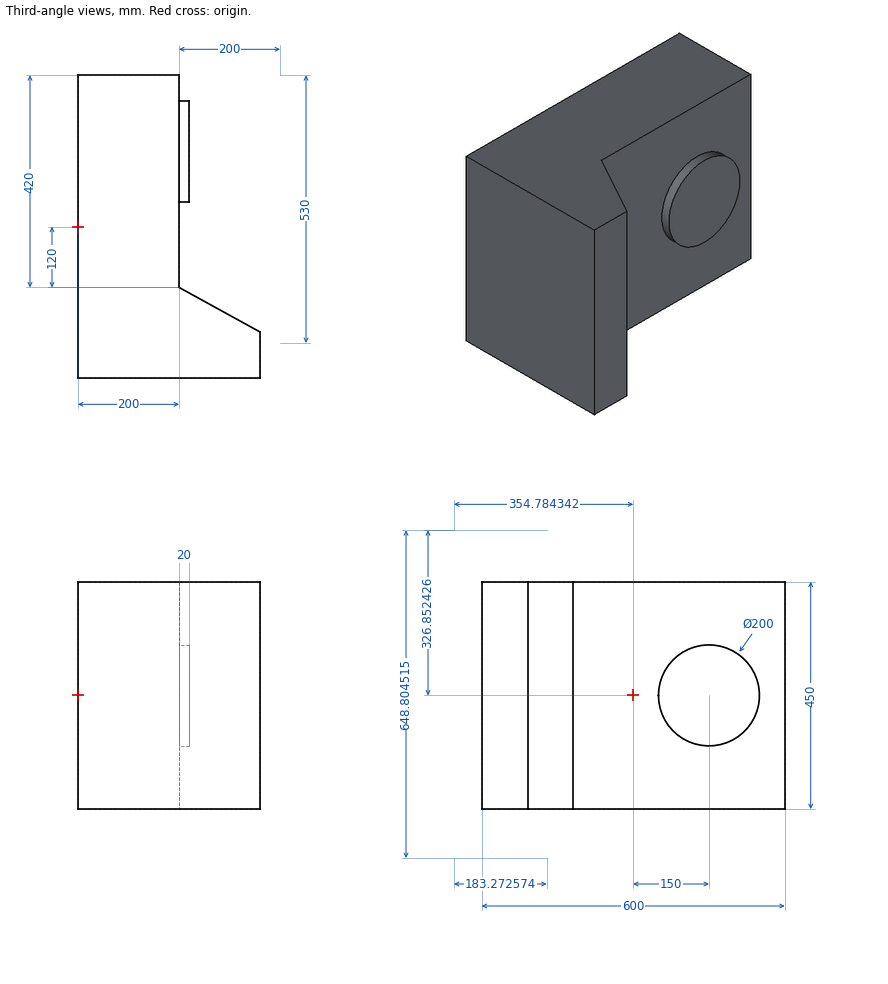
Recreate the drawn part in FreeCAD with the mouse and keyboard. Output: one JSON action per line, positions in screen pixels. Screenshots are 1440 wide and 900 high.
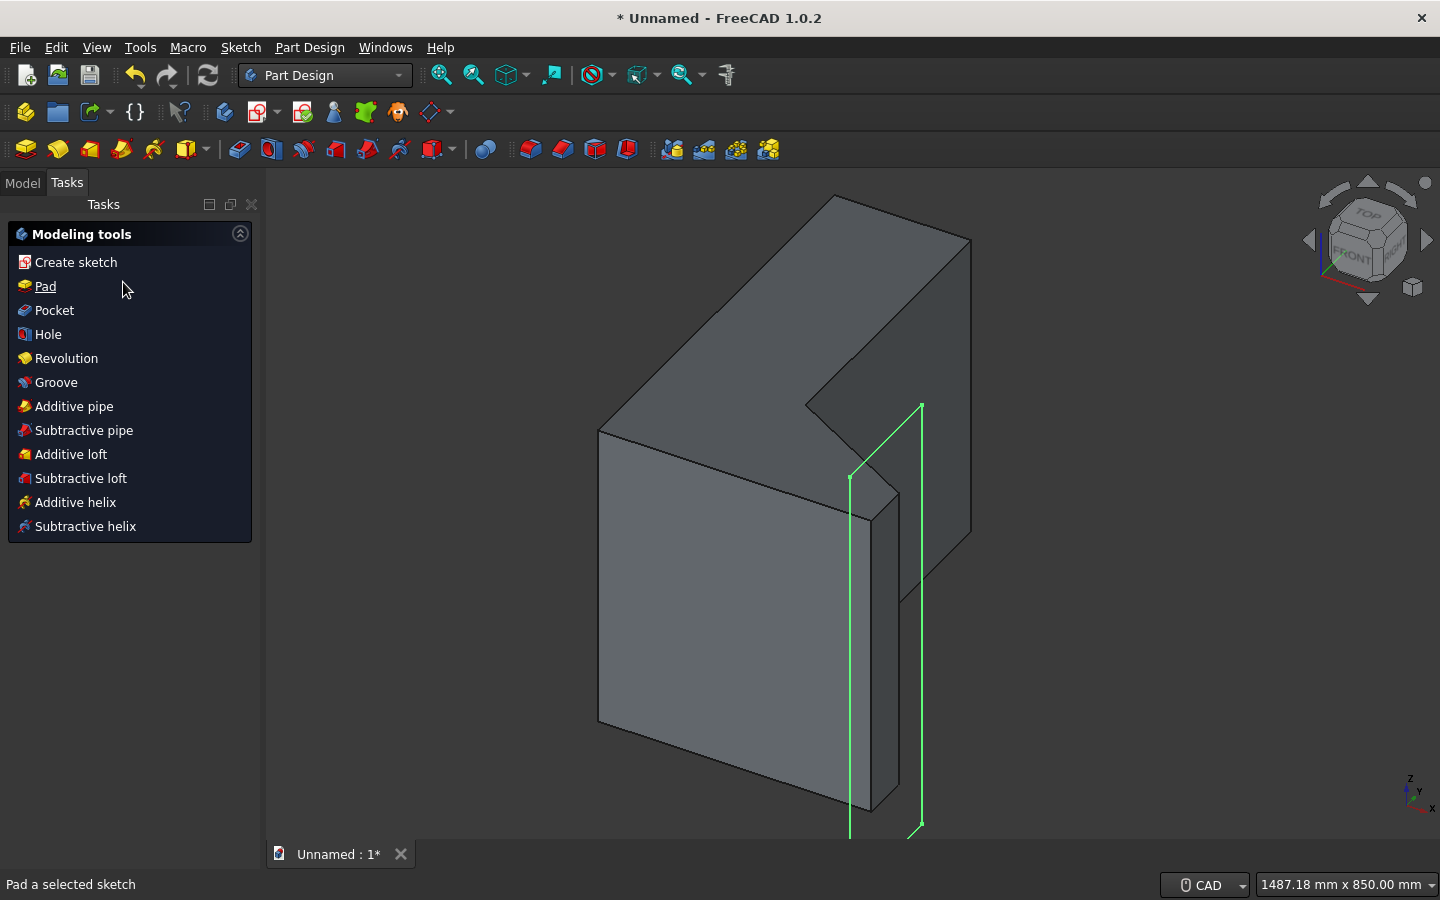
{"action": "left_click", "coordinate": [240, 150]}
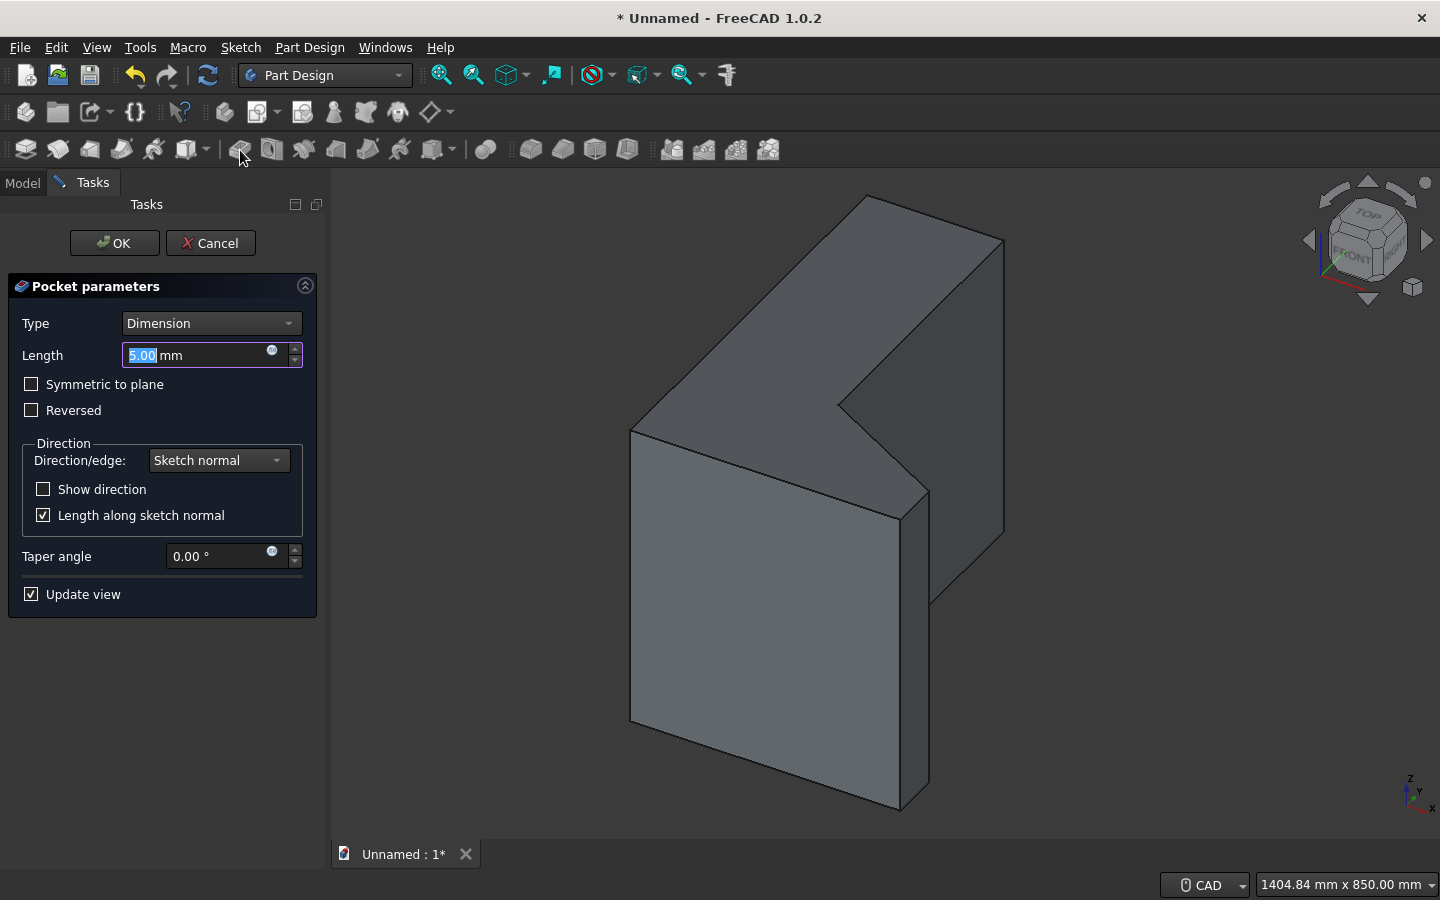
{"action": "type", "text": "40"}
{"action": "key", "text": "Tab"}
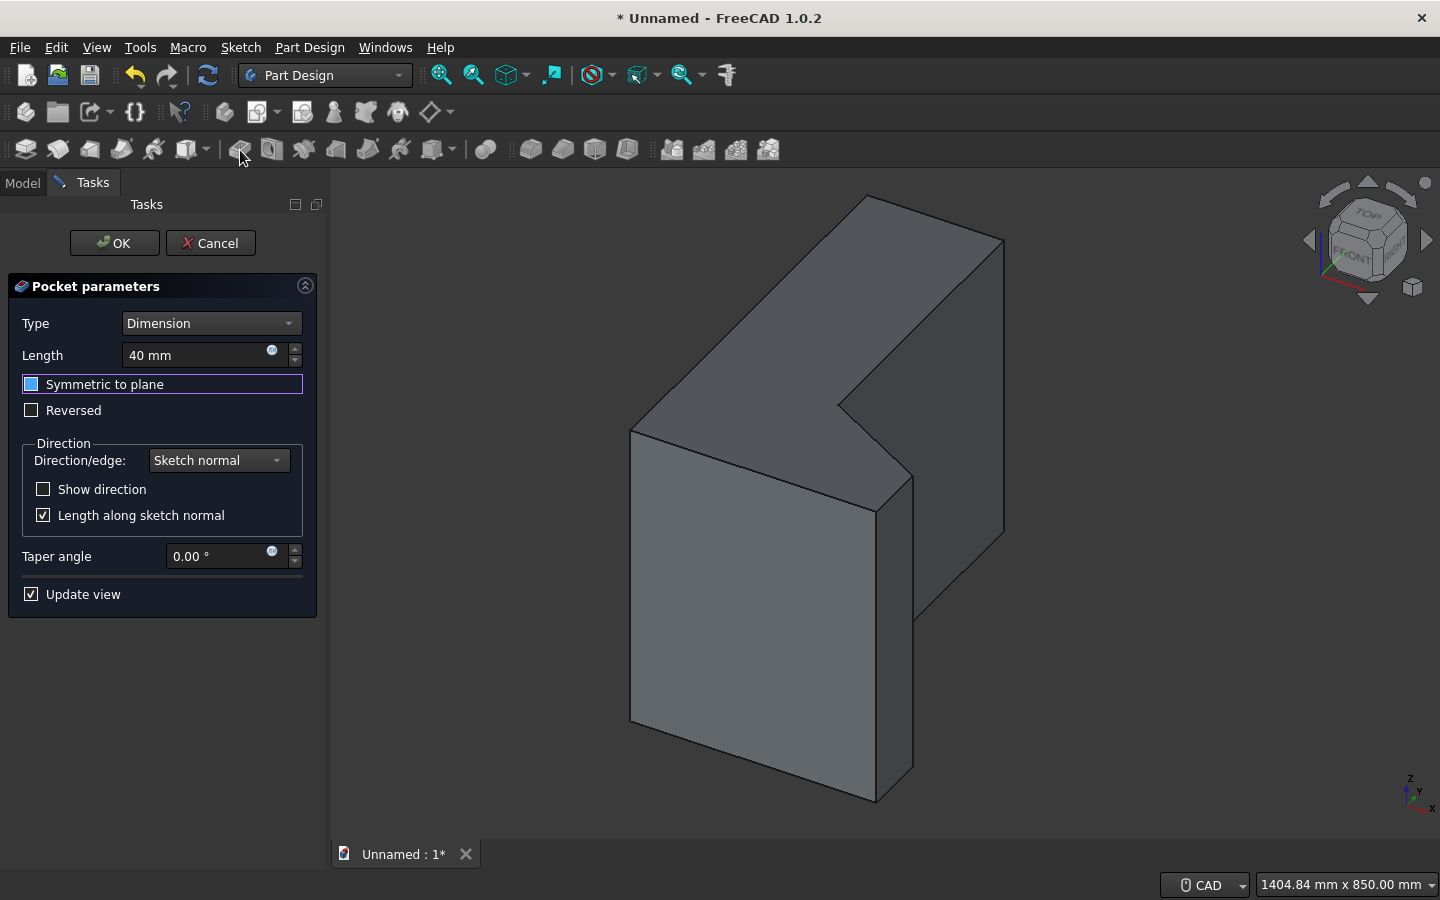
{"action": "left_click", "coordinate": [115, 243]}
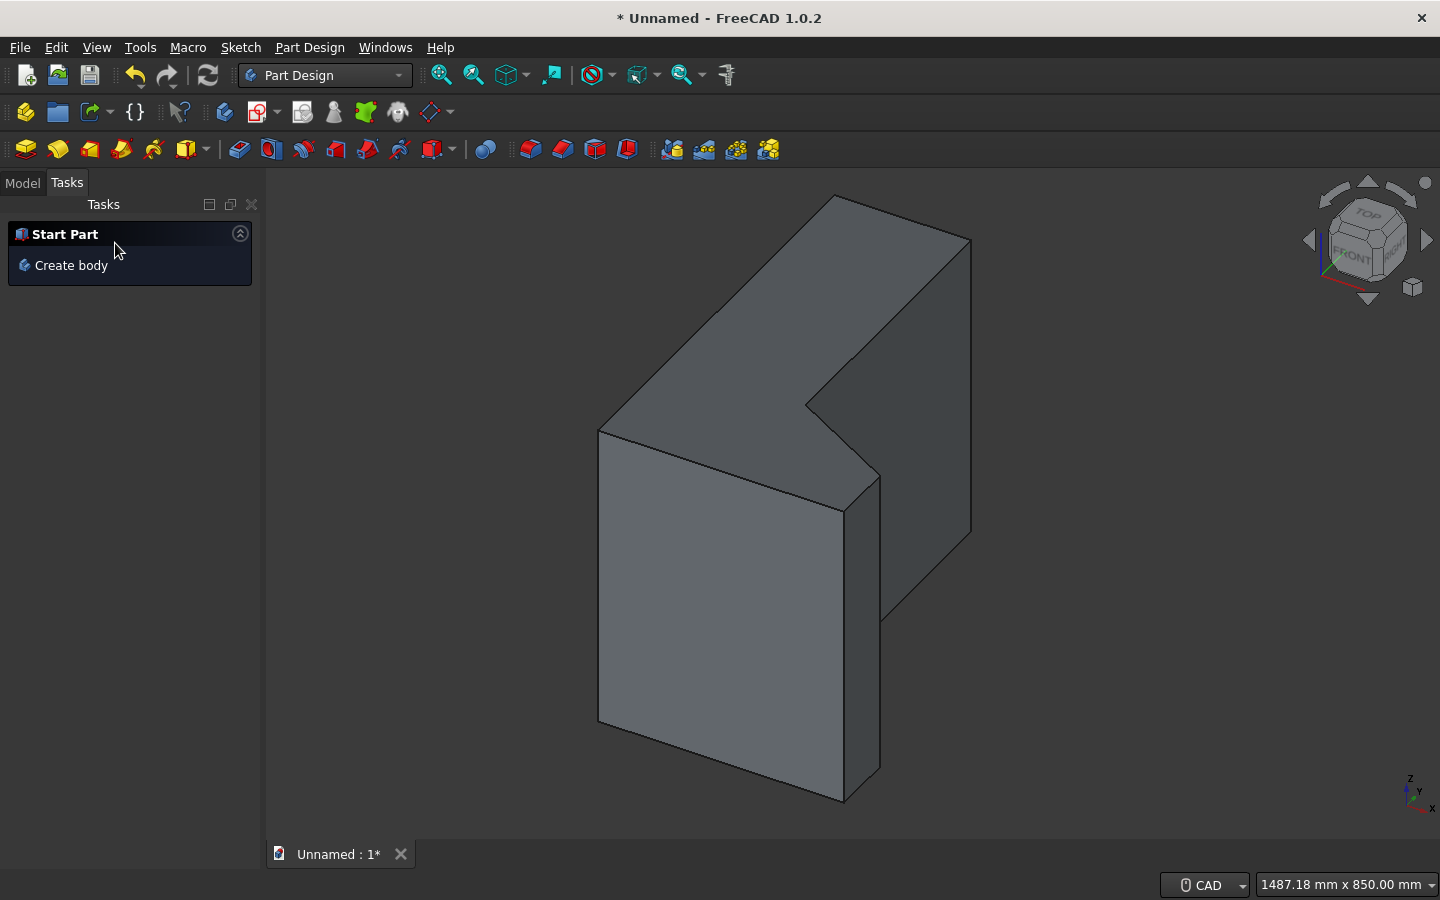
{"action": "left_click", "coordinate": [889, 467]}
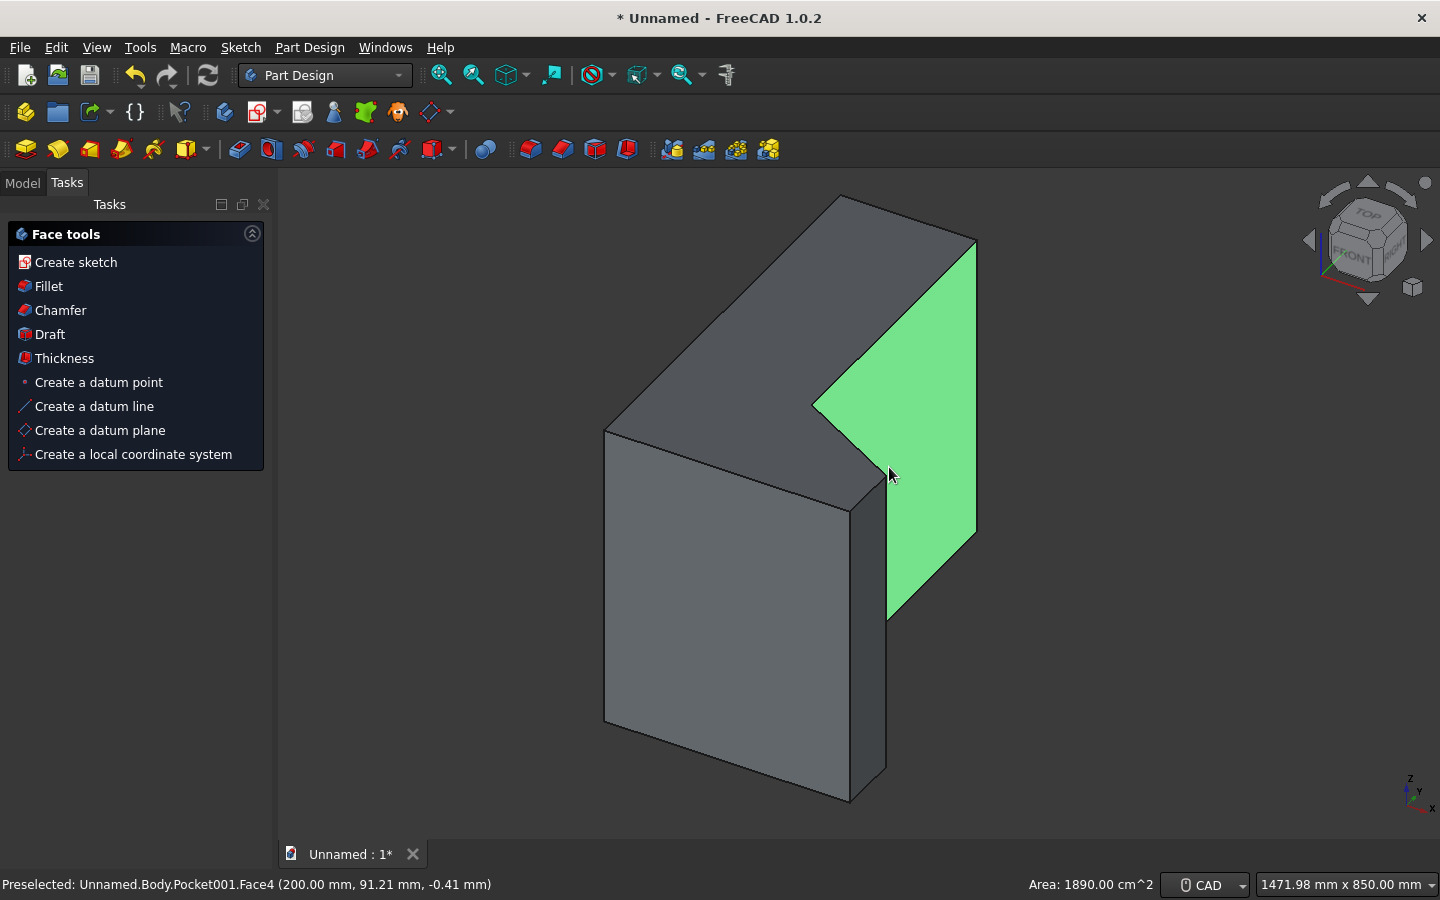
{"action": "left_click", "coordinate": [258, 112]}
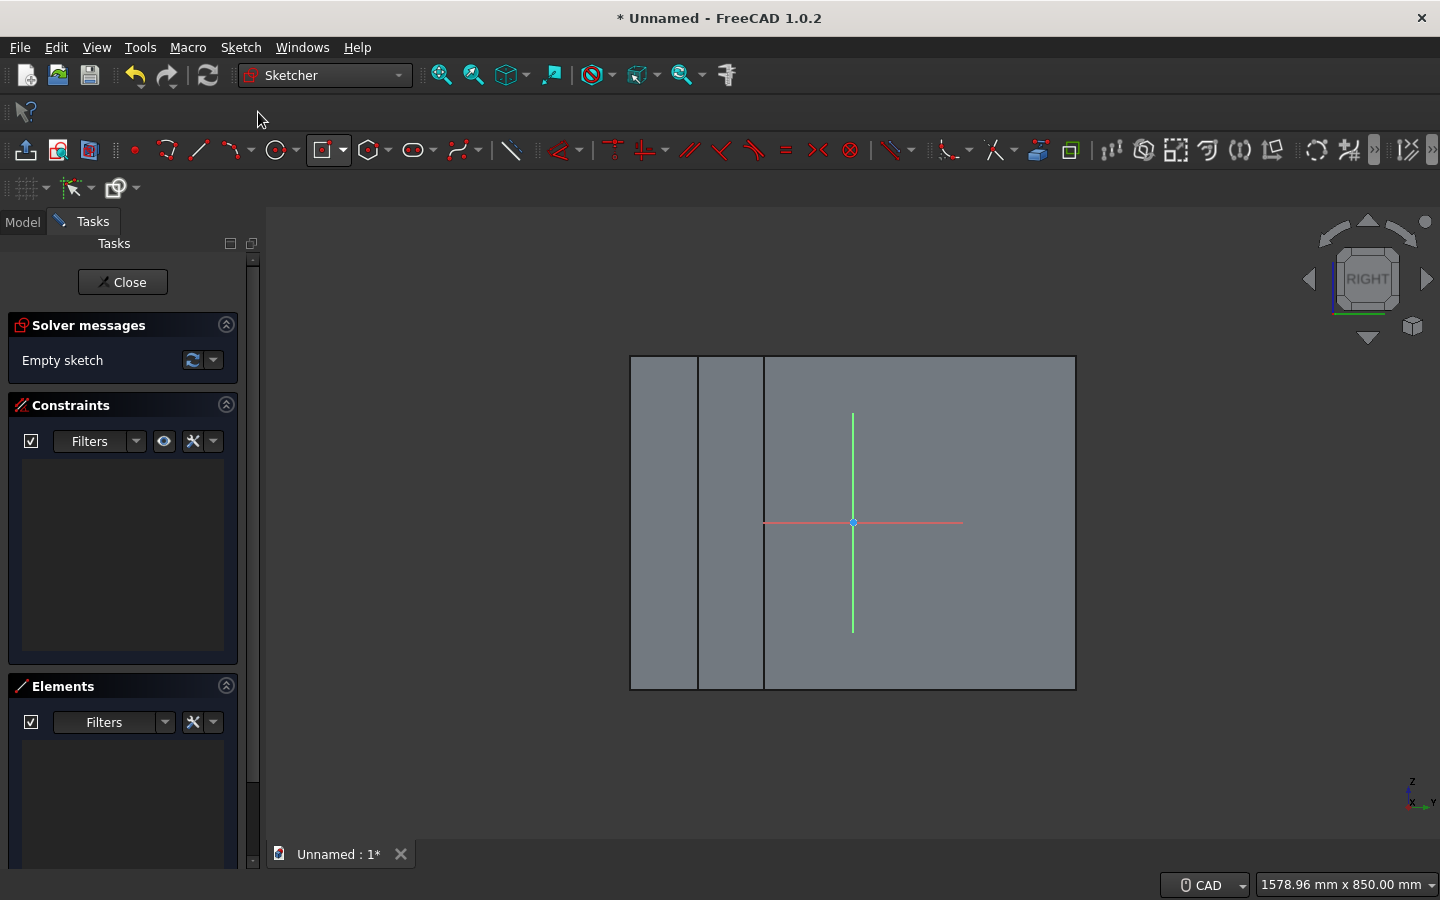
{"action": "scroll", "coordinate": [1040, 523], "scroll_direction": "up", "scroll_amount": 5}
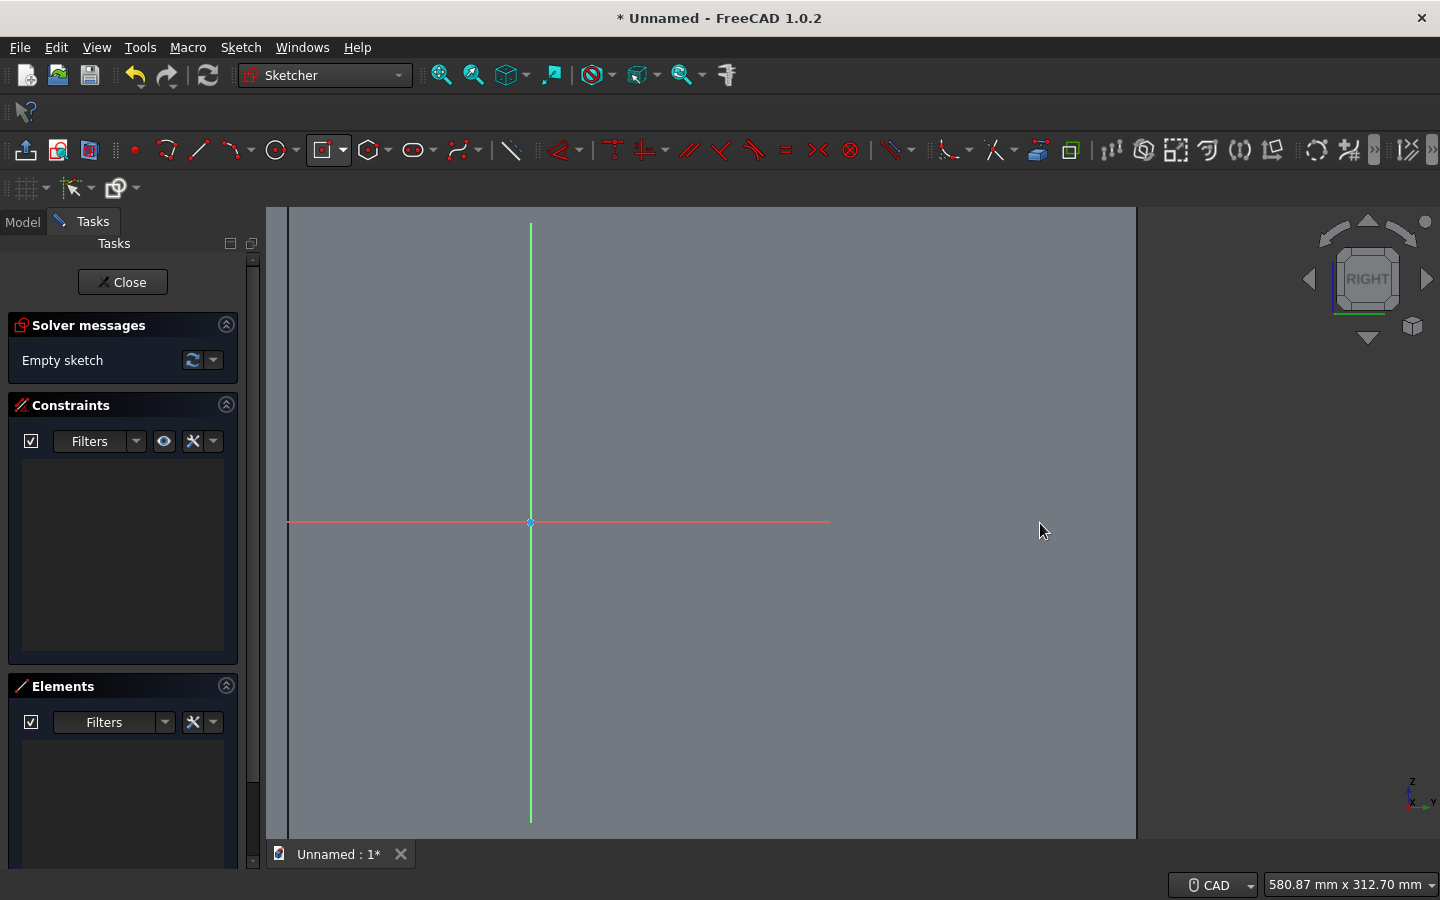
{"action": "key", "text": "g c"}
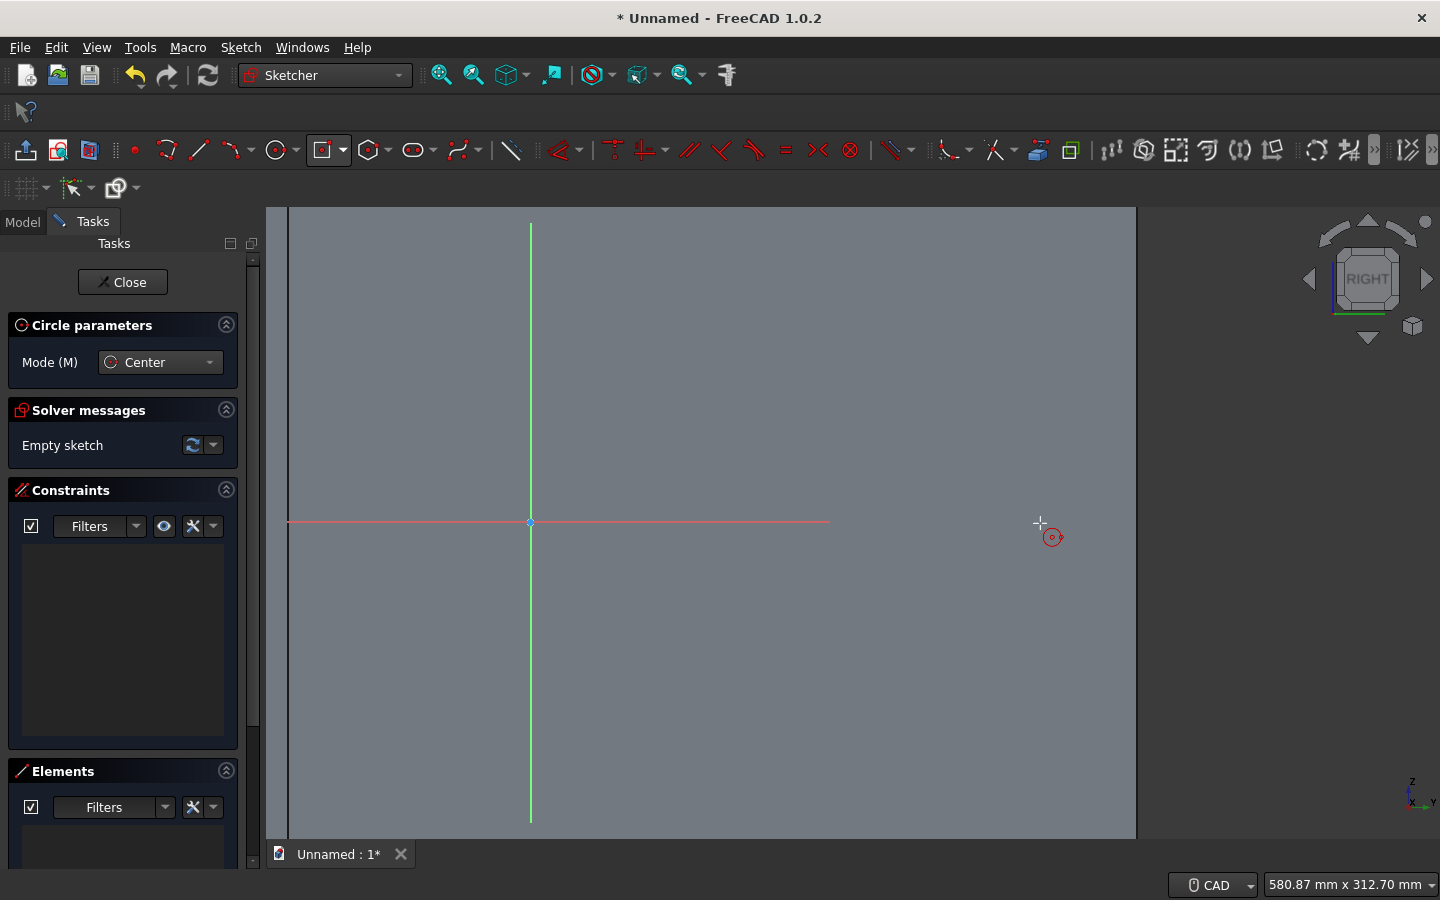
{"action": "left_click", "coordinate": [834, 522]}
{"action": "mouse_move", "coordinate": [977, 379]}